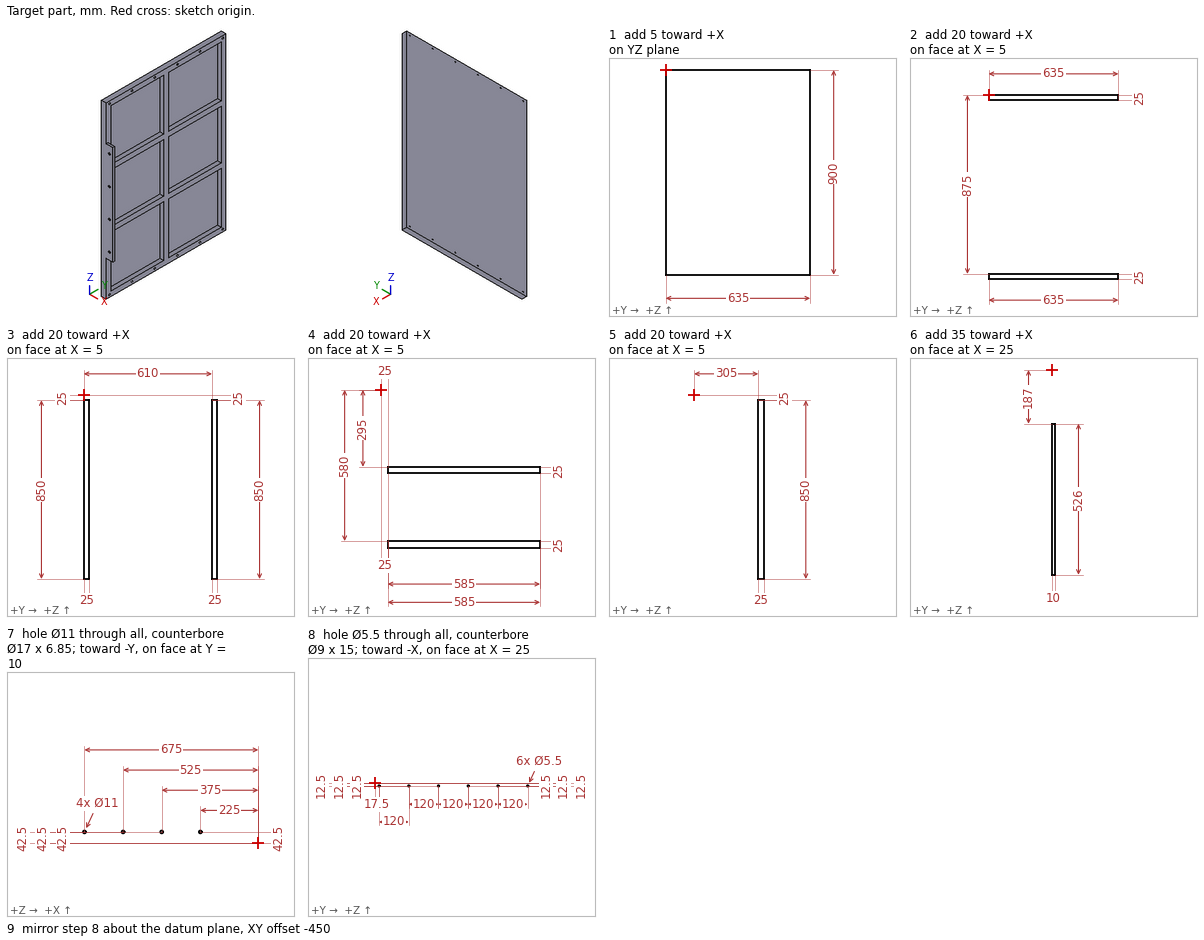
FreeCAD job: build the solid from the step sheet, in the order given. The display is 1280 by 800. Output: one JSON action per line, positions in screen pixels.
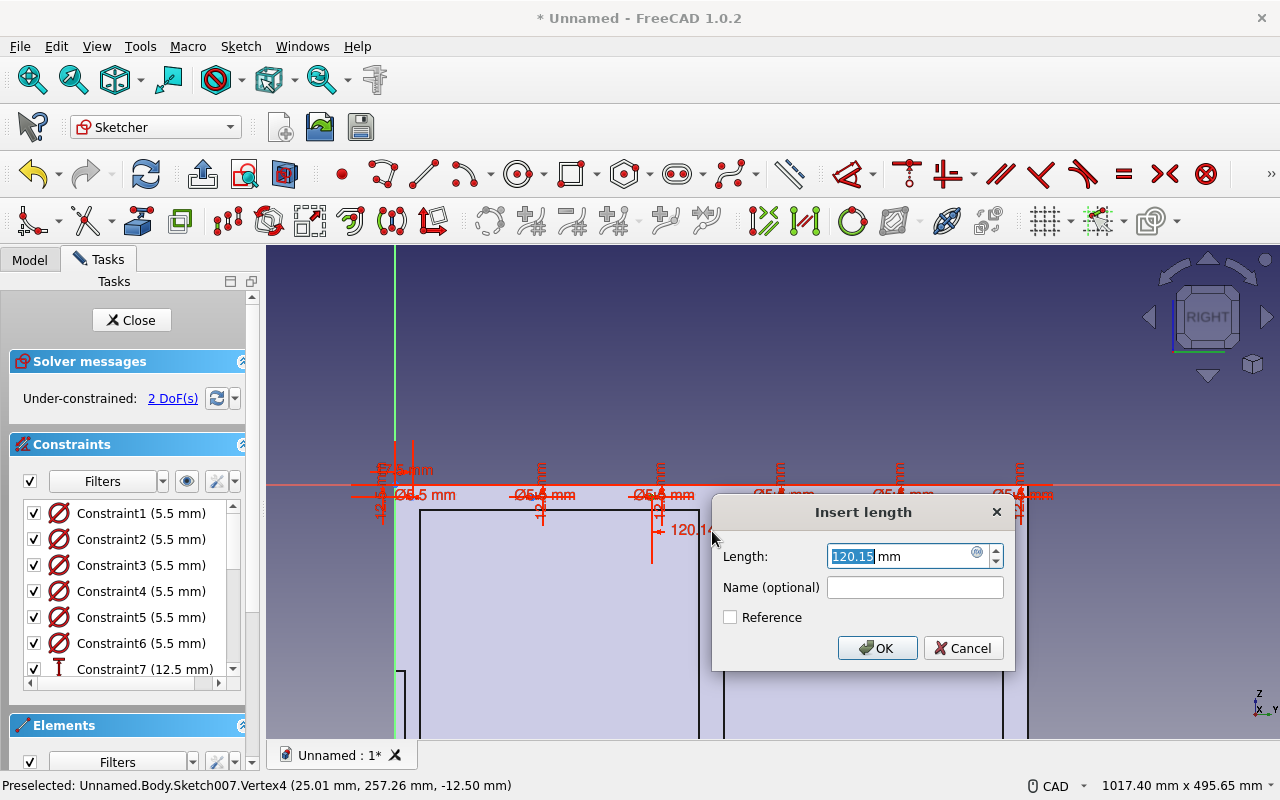
{"action": "type", "text": "120"}
{"action": "key", "text": "Return"}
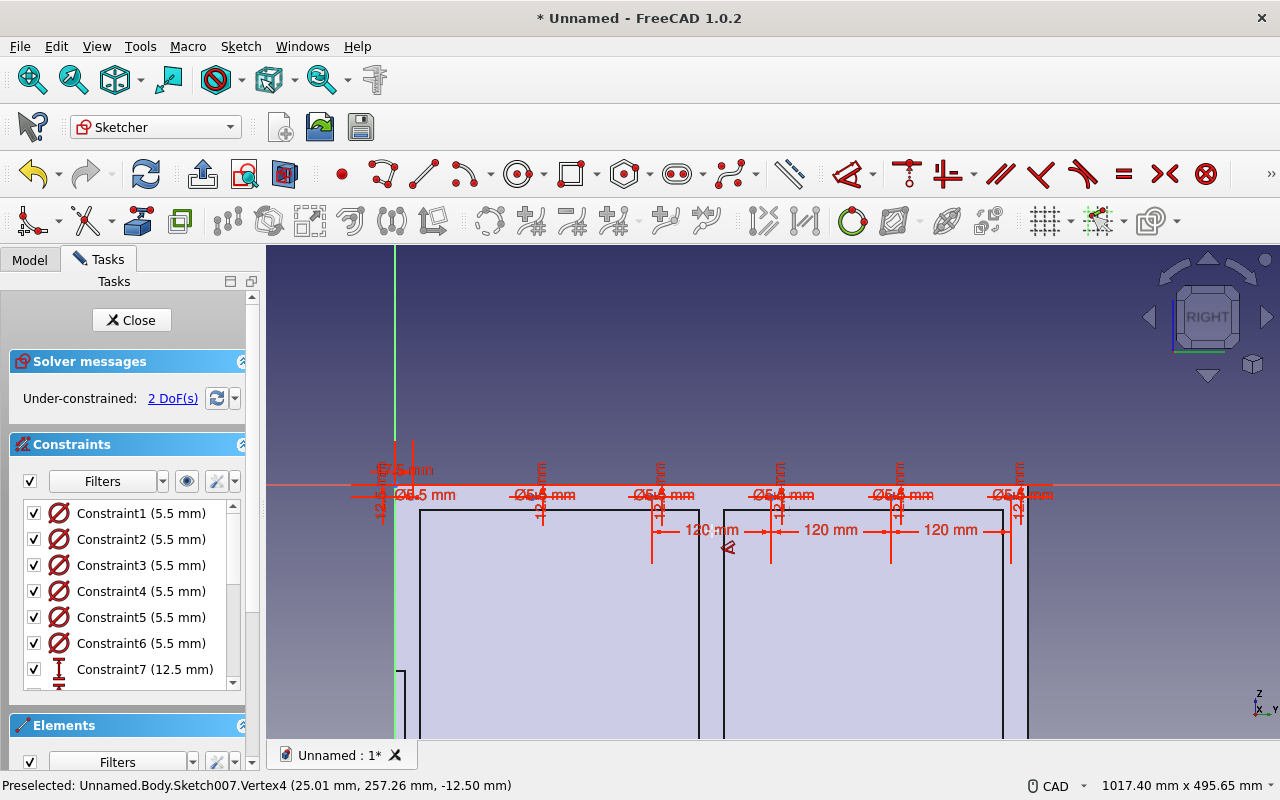
{"action": "left_click", "coordinate": [652, 497]}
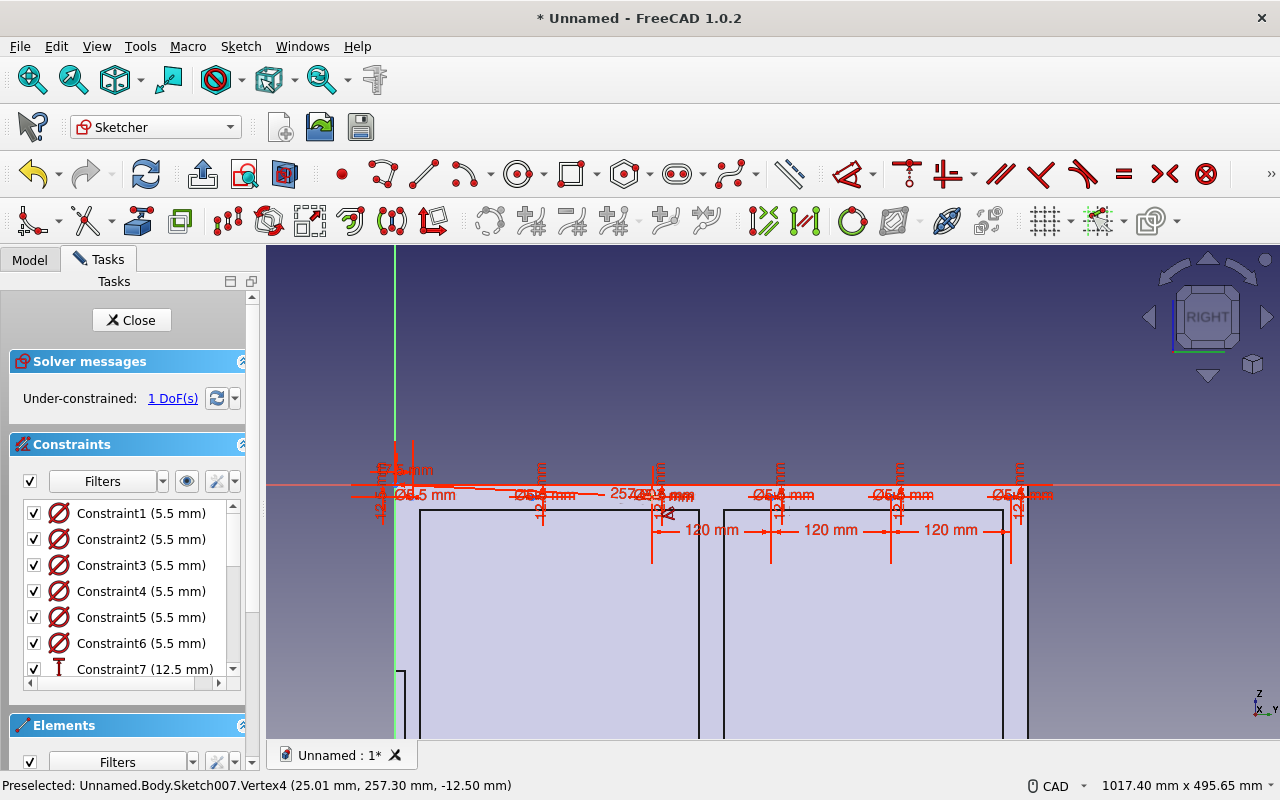
{"action": "left_click", "coordinate": [533, 497]}
{"action": "left_click", "coordinate": [592, 531]}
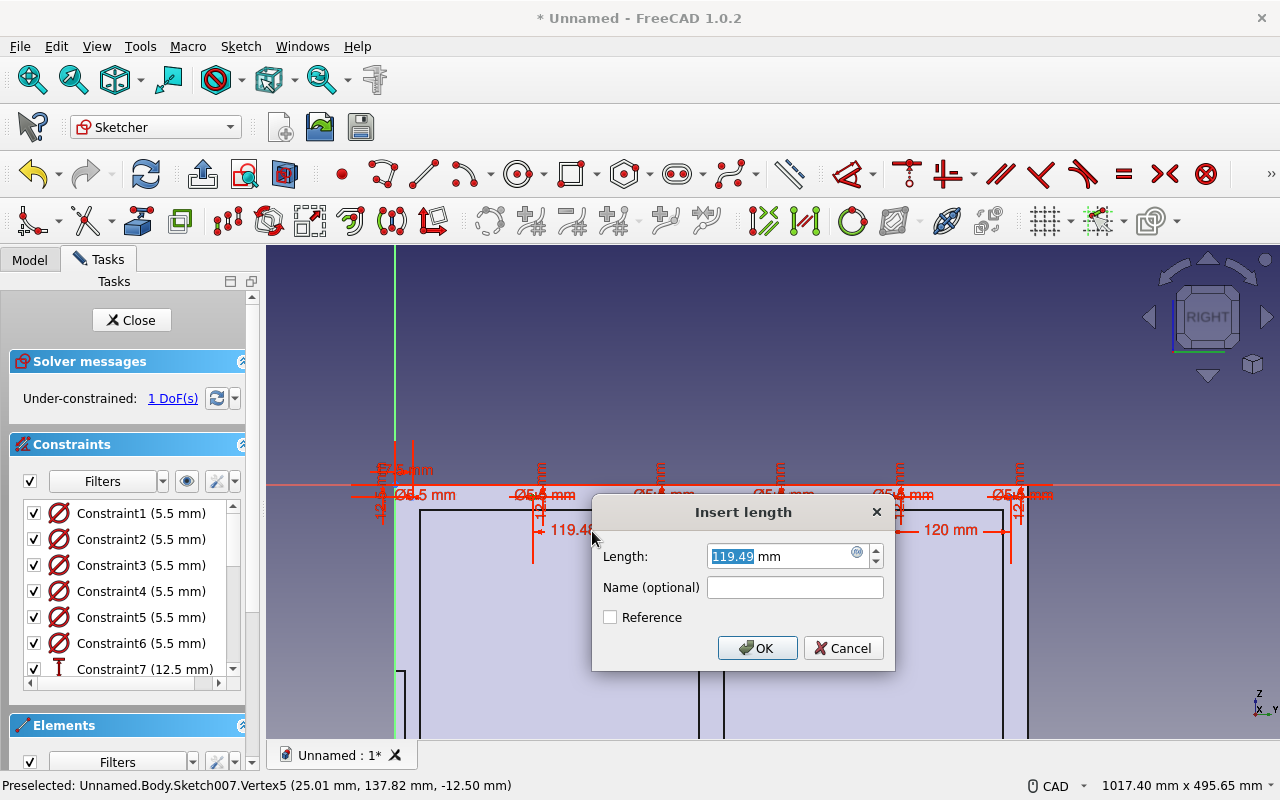
{"action": "type", "text": "120"}
{"action": "key", "text": "Return"}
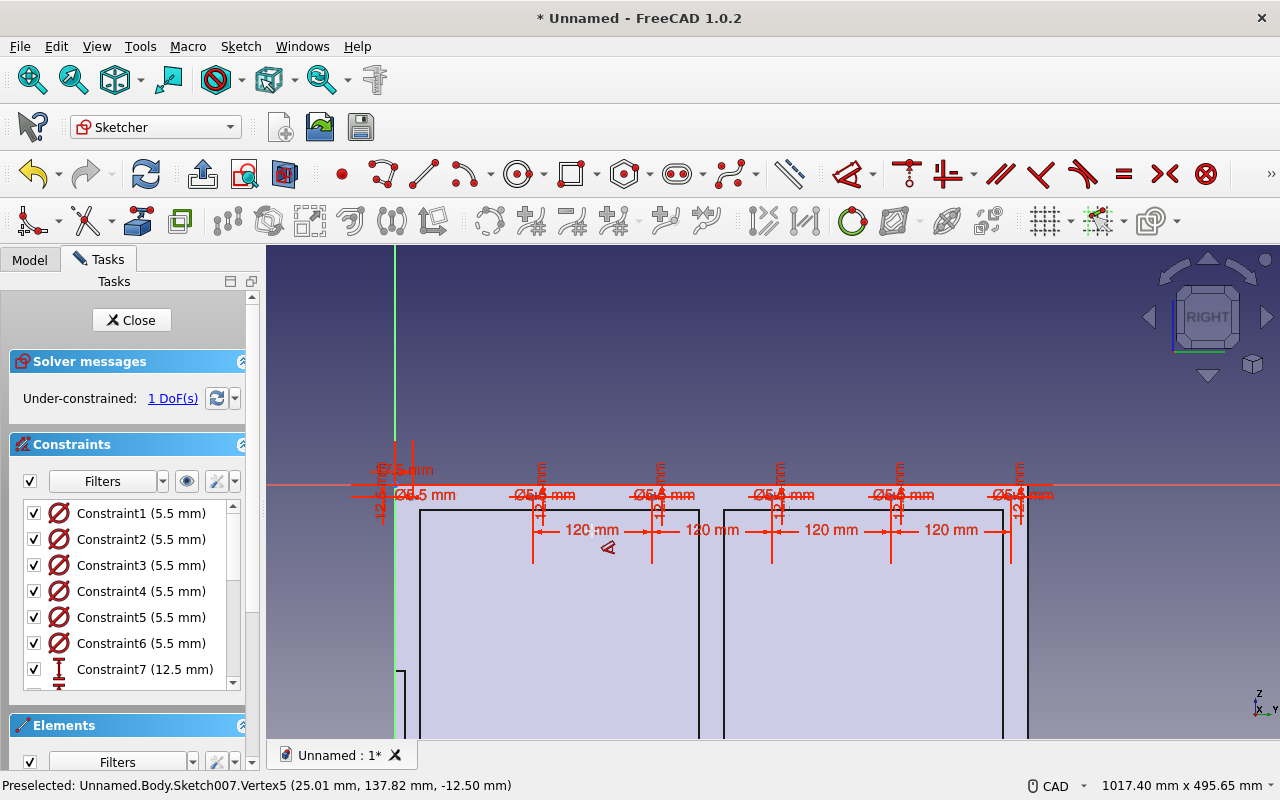
{"action": "left_click", "coordinate": [533, 497]}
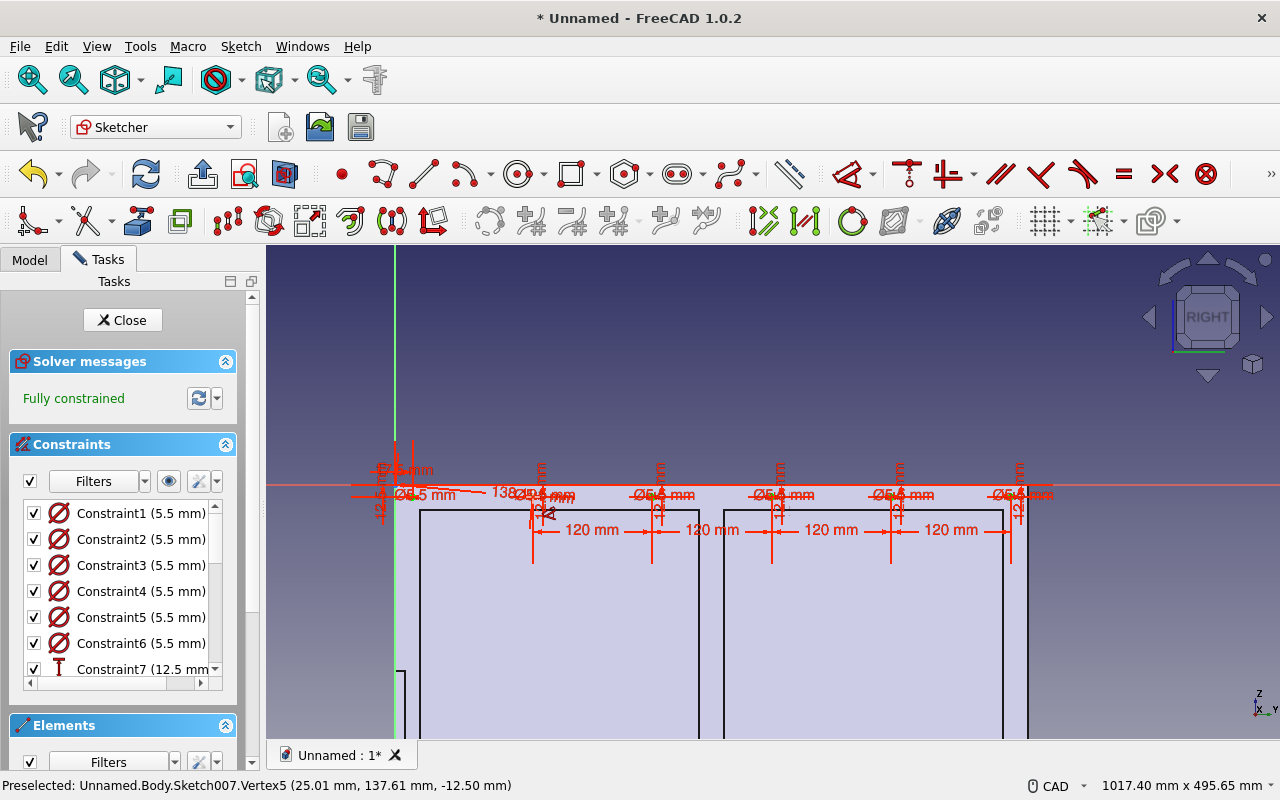
{"action": "left_click", "coordinate": [413, 497]}
{"action": "left_click", "coordinate": [473, 531]}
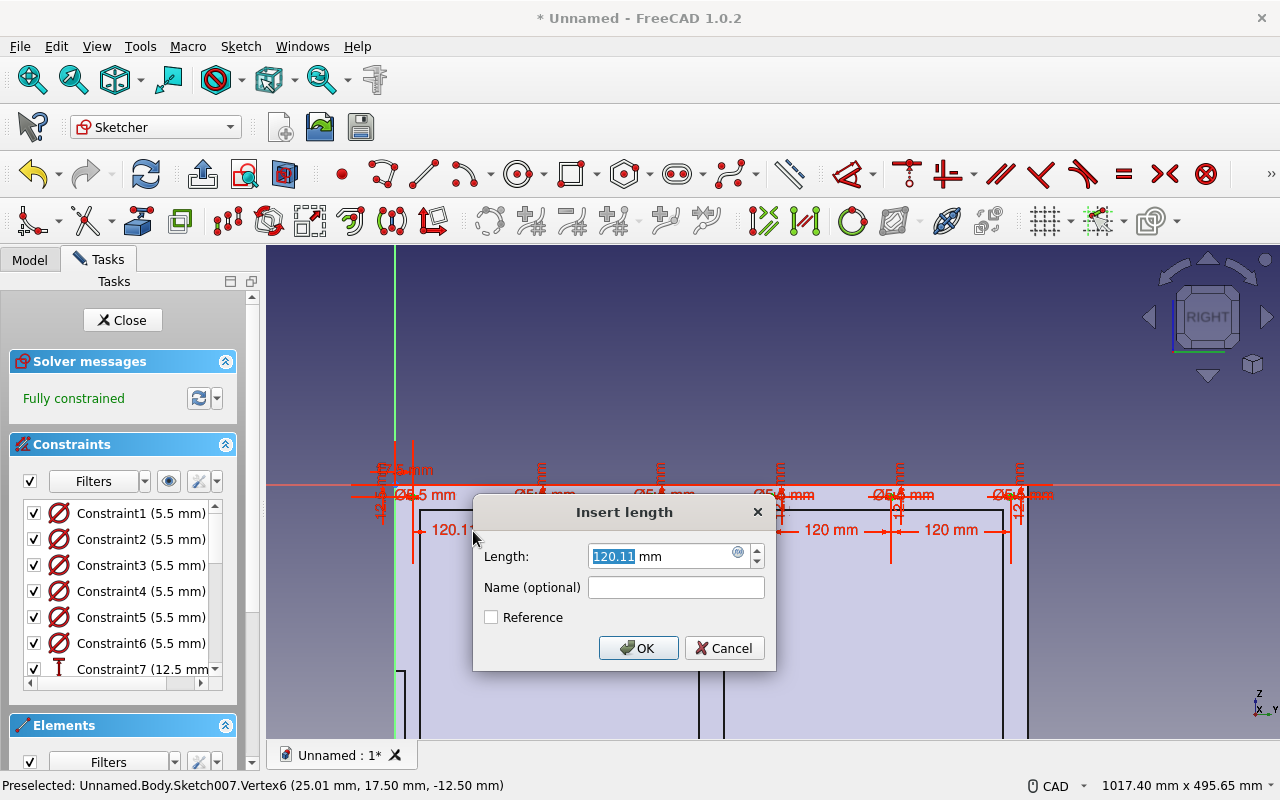
{"action": "type", "text": "120"}
{"action": "key", "text": "Return"}
{"action": "key", "text": "Escape"}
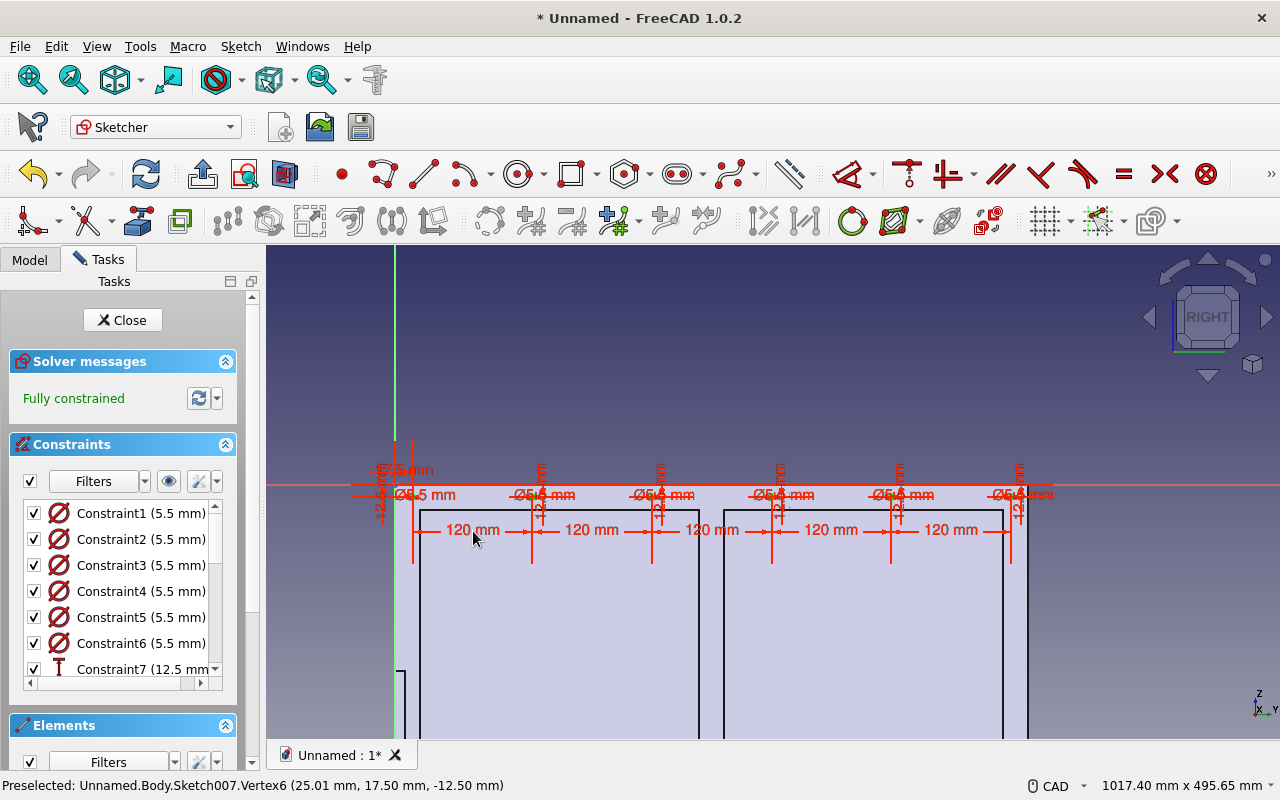
{"action": "left_click", "coordinate": [123, 320]}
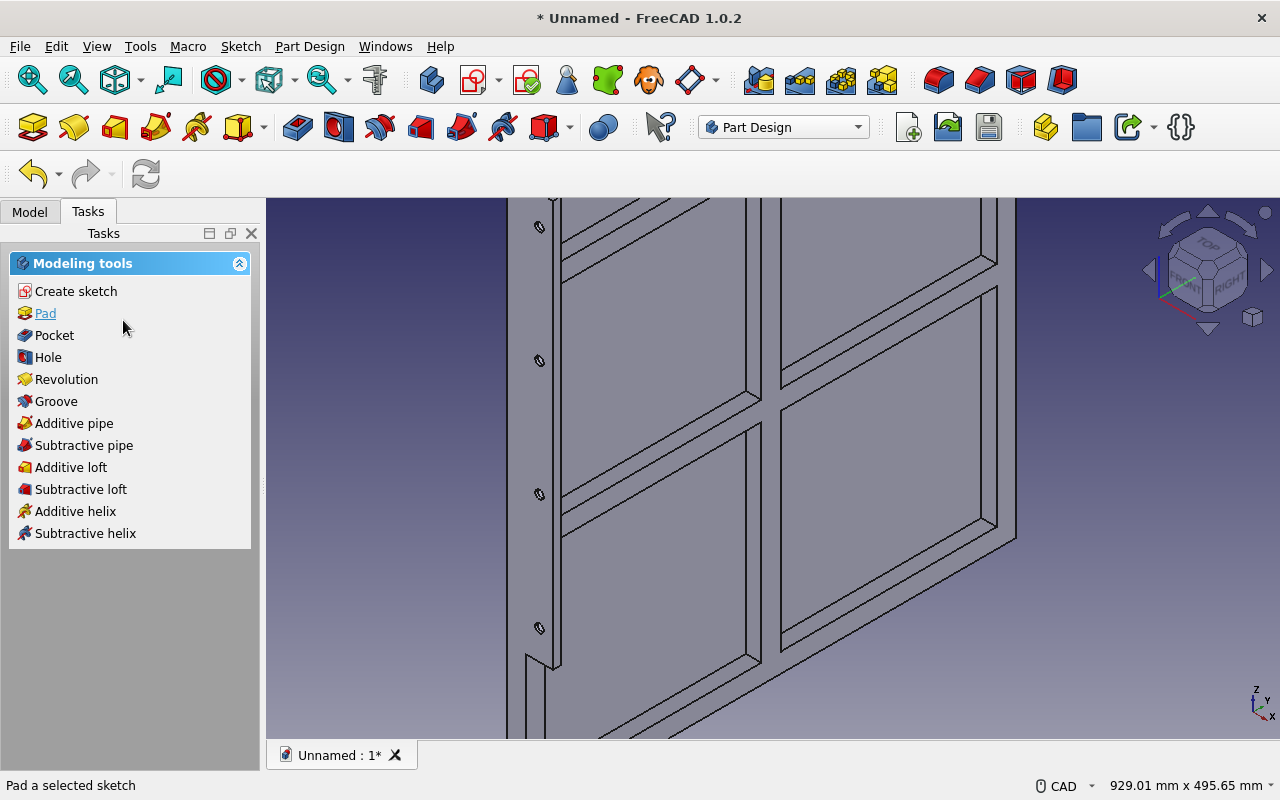
{"action": "left_click", "coordinate": [339, 128]}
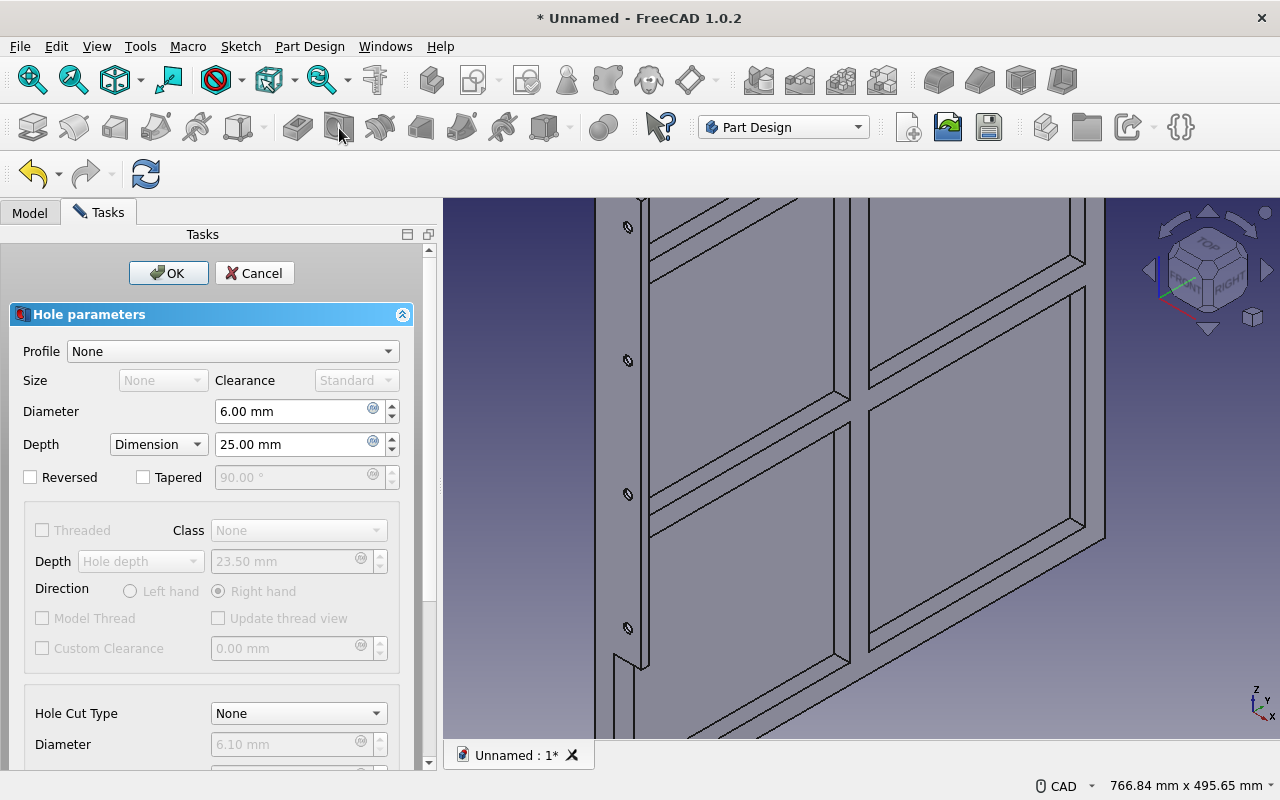
{"action": "triple_click", "coordinate": [300, 412]}